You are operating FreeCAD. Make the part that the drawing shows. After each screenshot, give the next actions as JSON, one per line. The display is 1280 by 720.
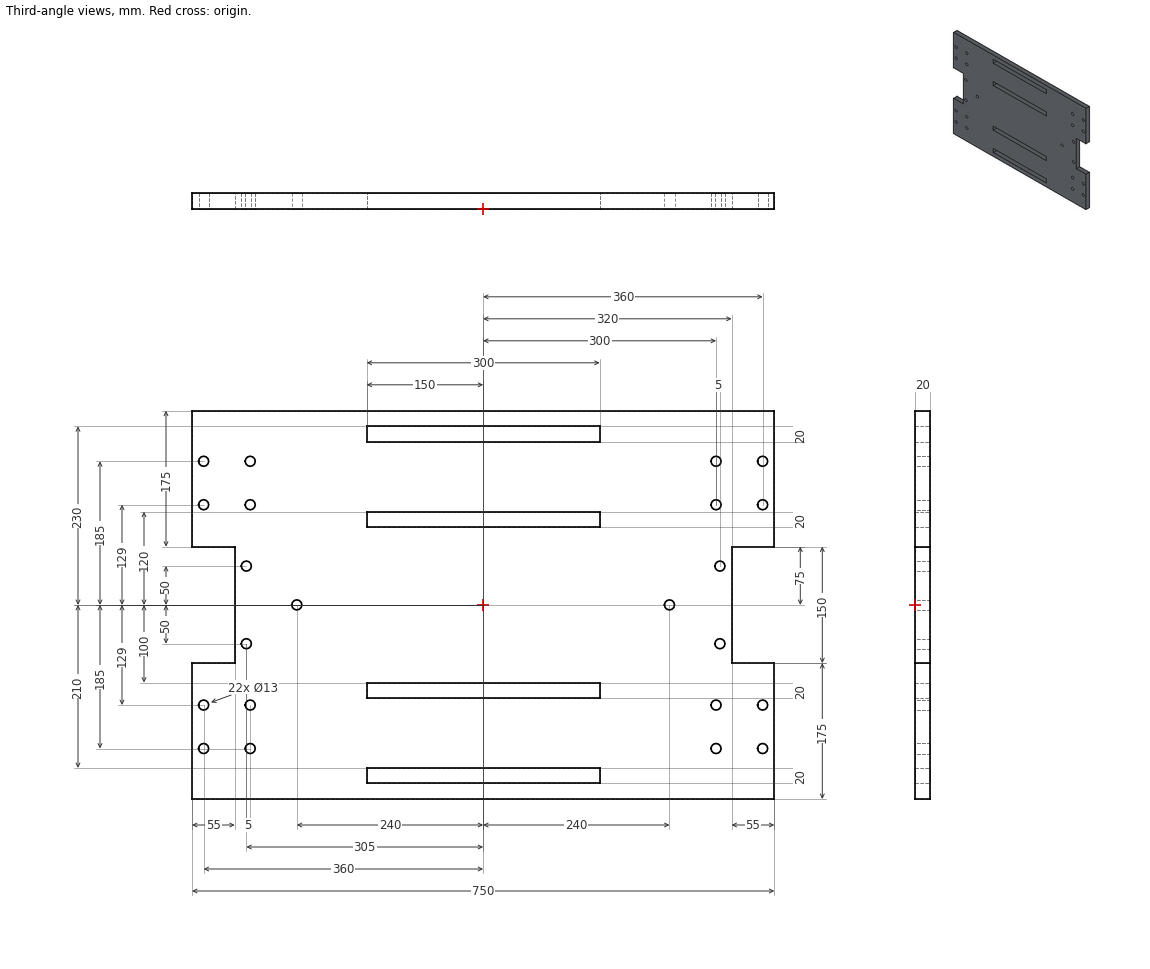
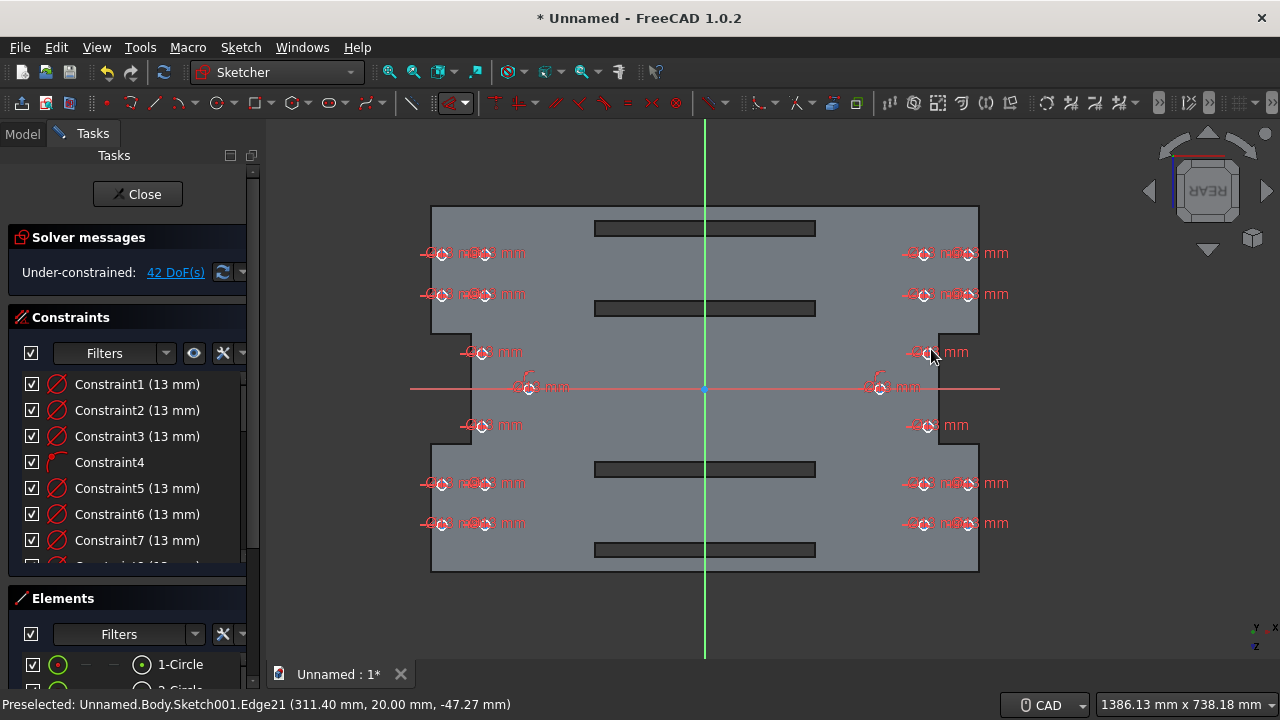
{"action": "left_click", "coordinate": [442, 296]}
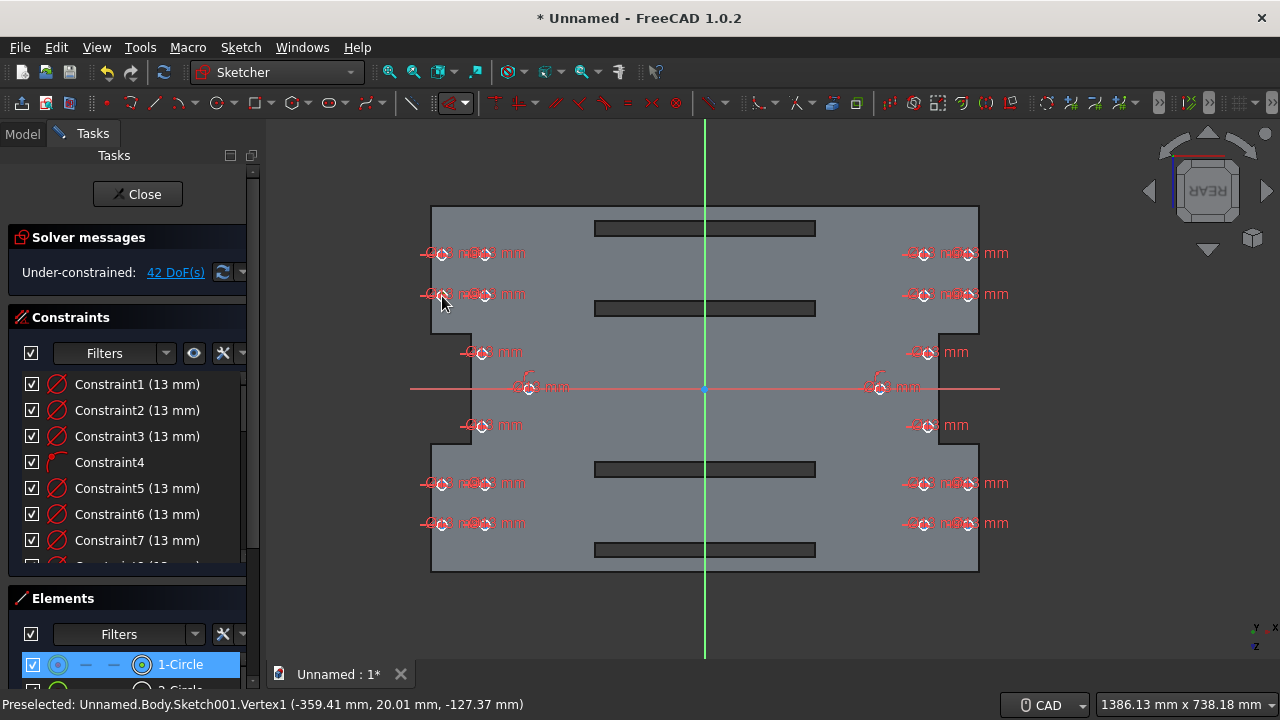
{"action": "left_click", "coordinate": [485, 296]}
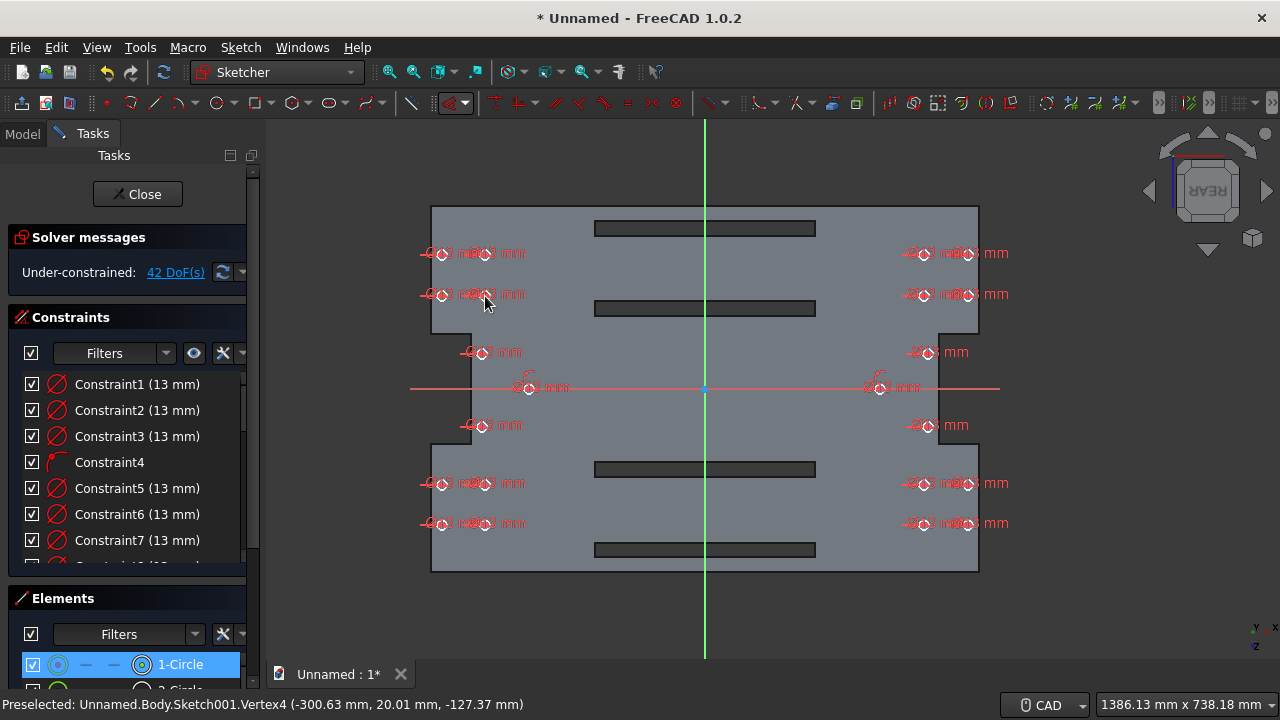
{"action": "left_click", "coordinate": [538, 104]}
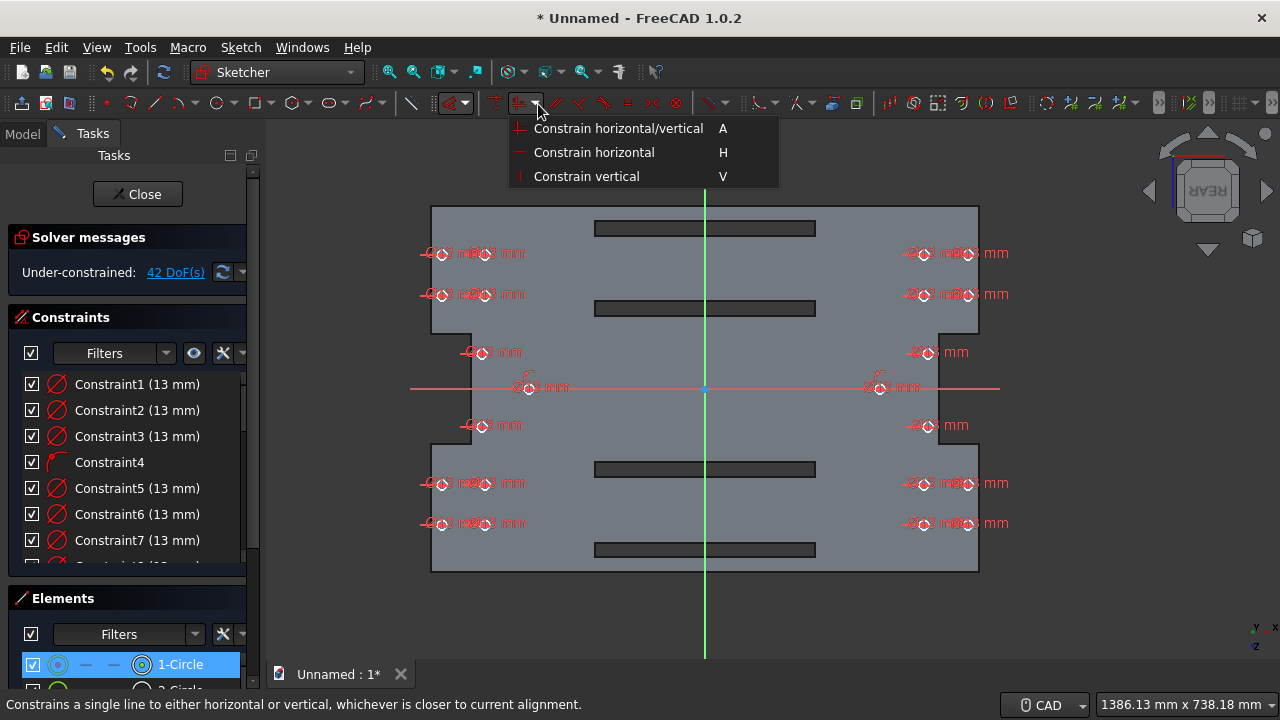
{"action": "left_click", "coordinate": [644, 152]}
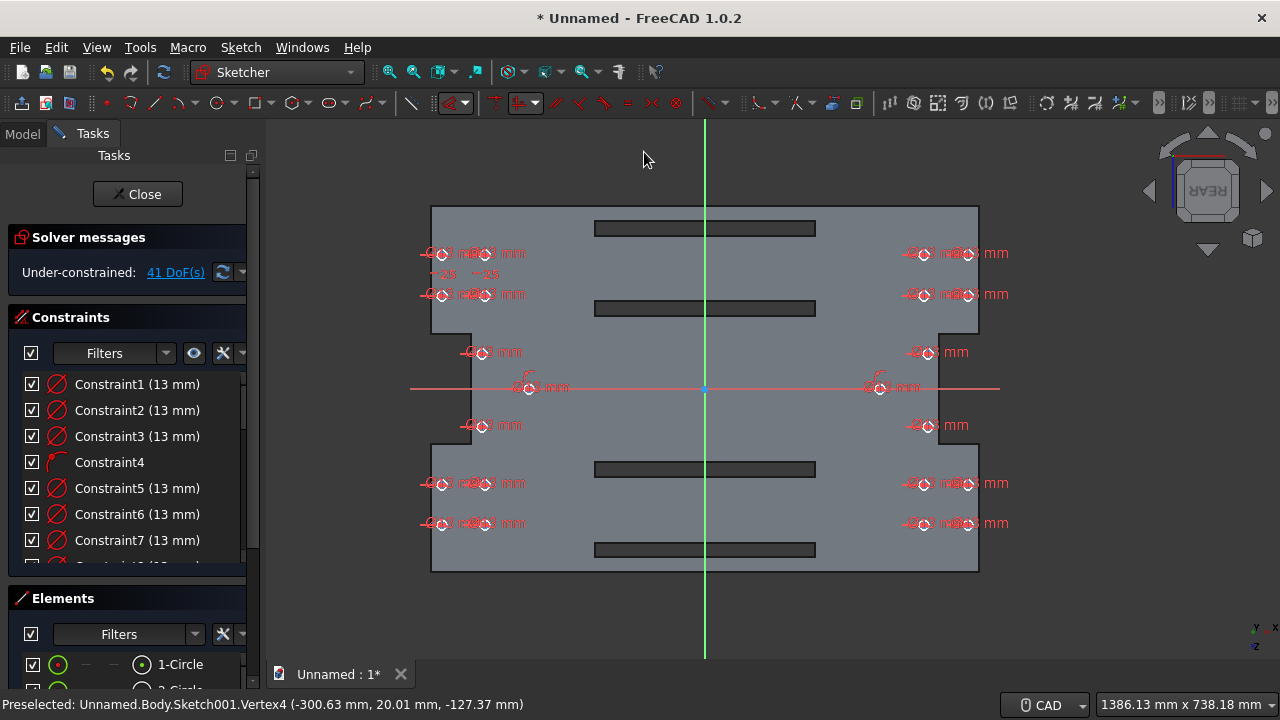
{"action": "left_click", "coordinate": [485, 296]}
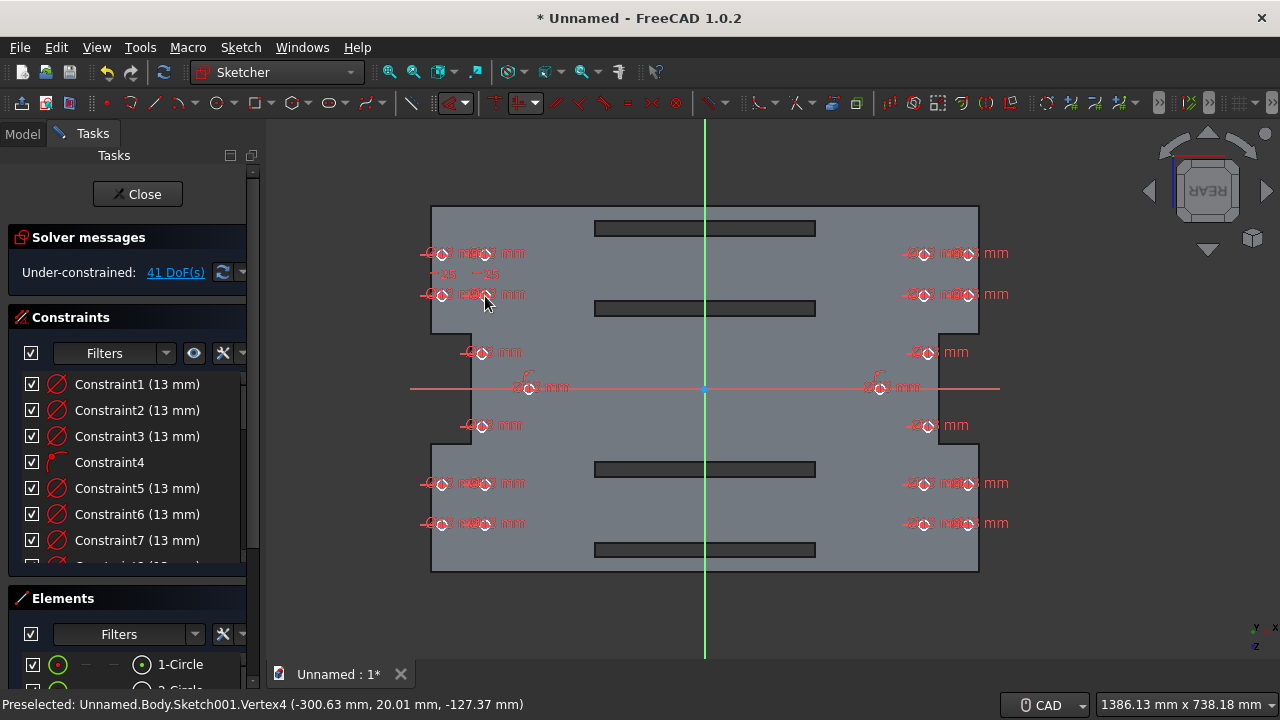
{"action": "left_click", "coordinate": [485, 255]}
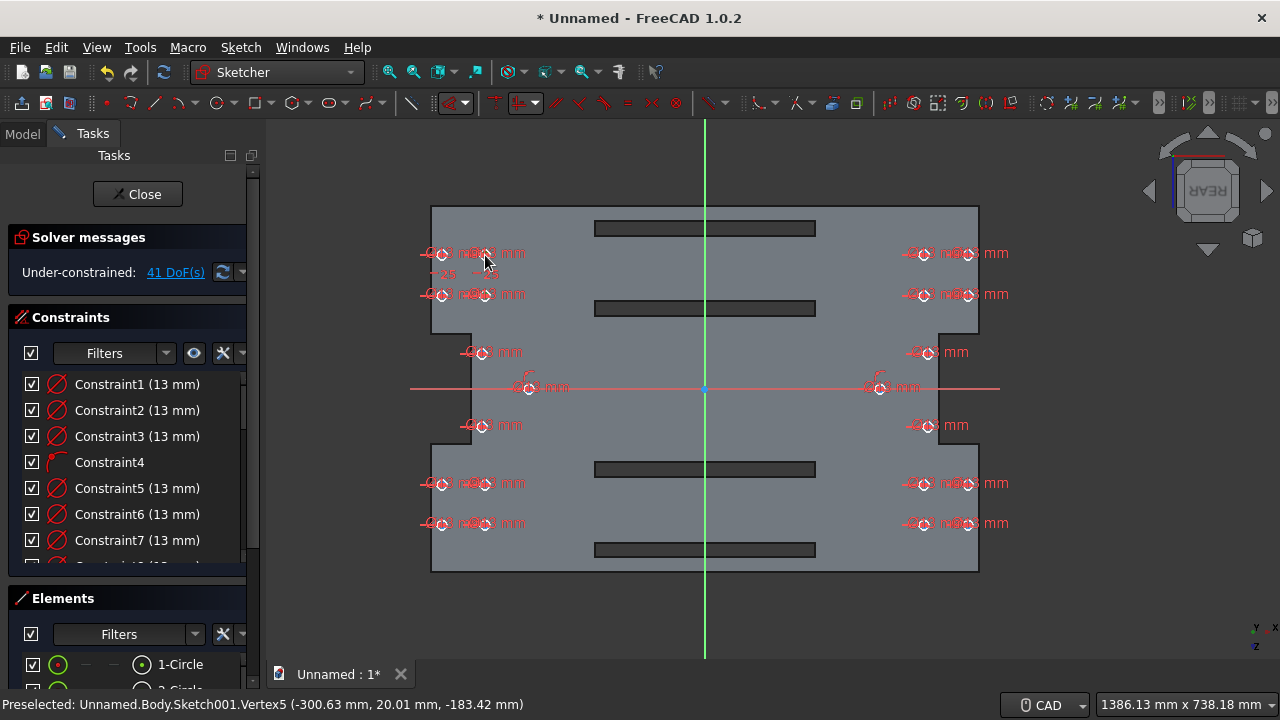
{"action": "key", "text": "v"}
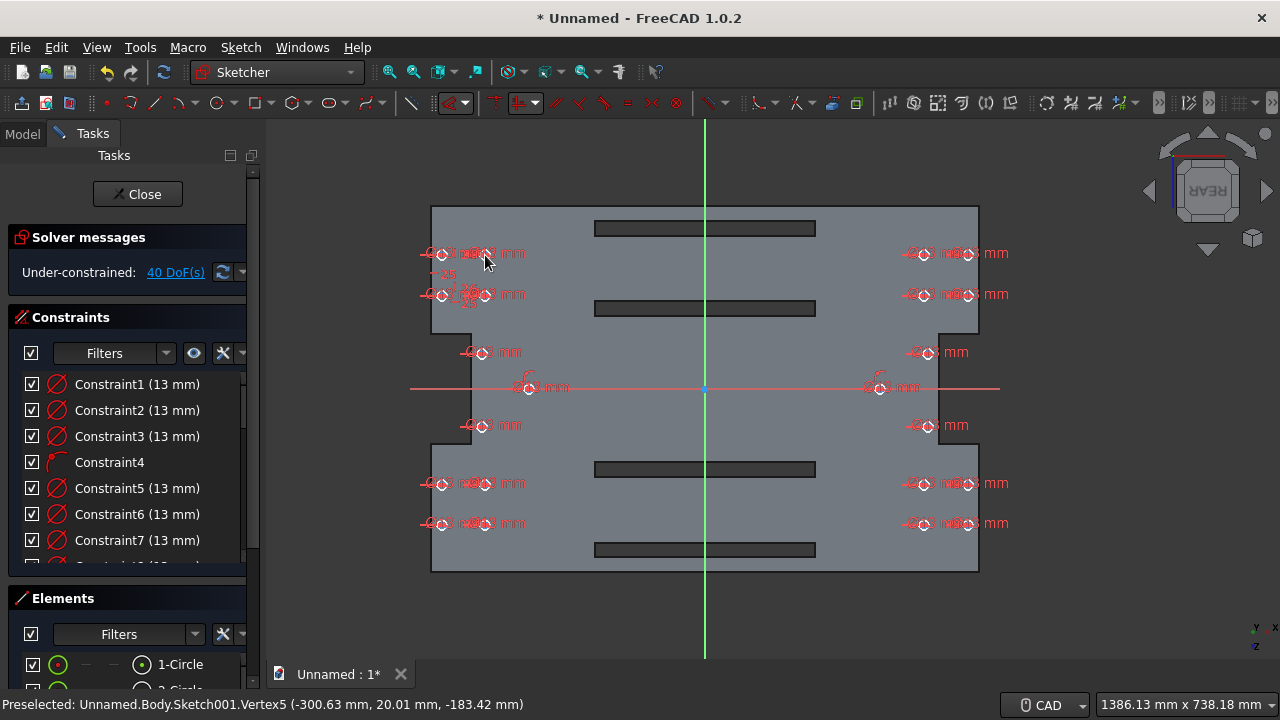
{"action": "left_click", "coordinate": [442, 296]}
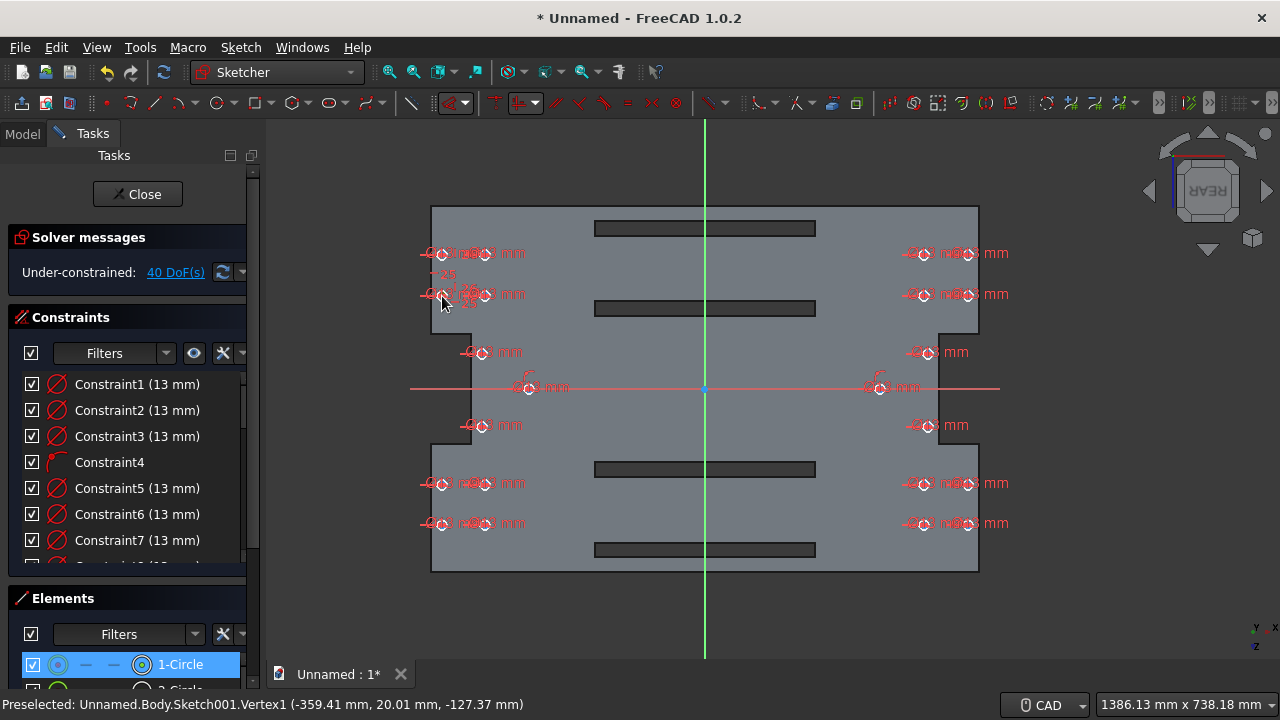
{"action": "left_click", "coordinate": [442, 255]}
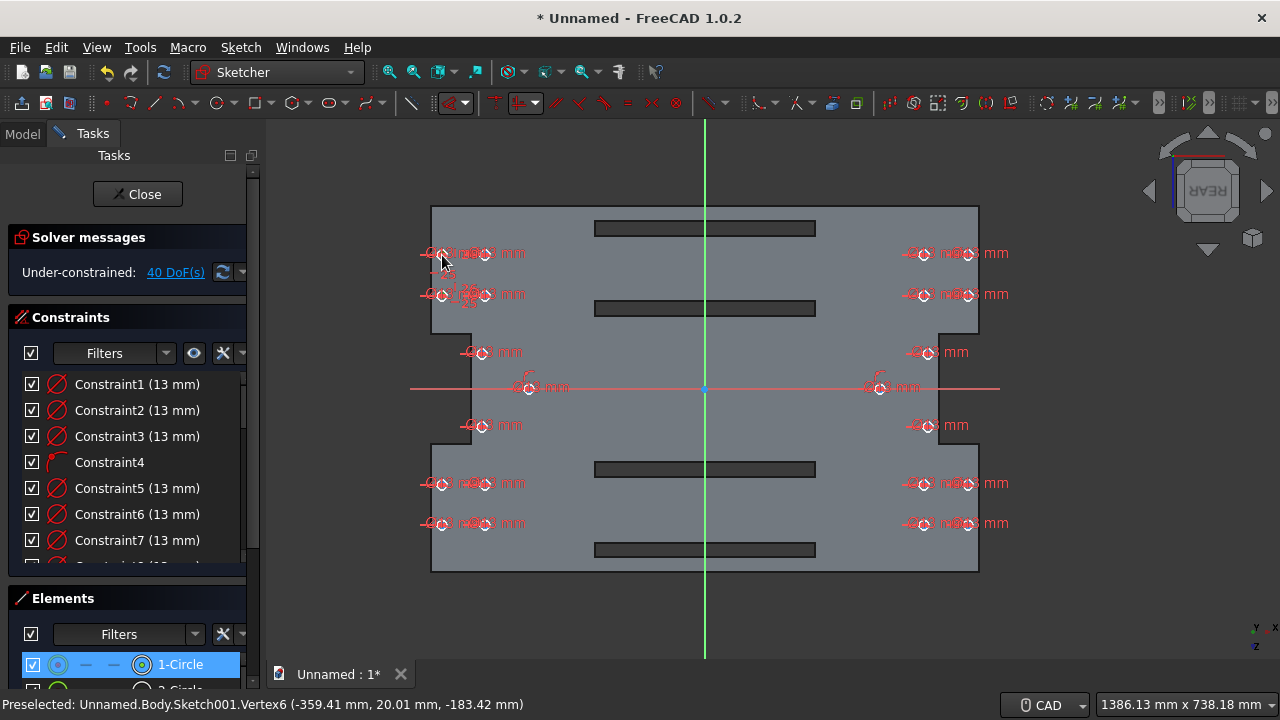
{"action": "key", "text": "v"}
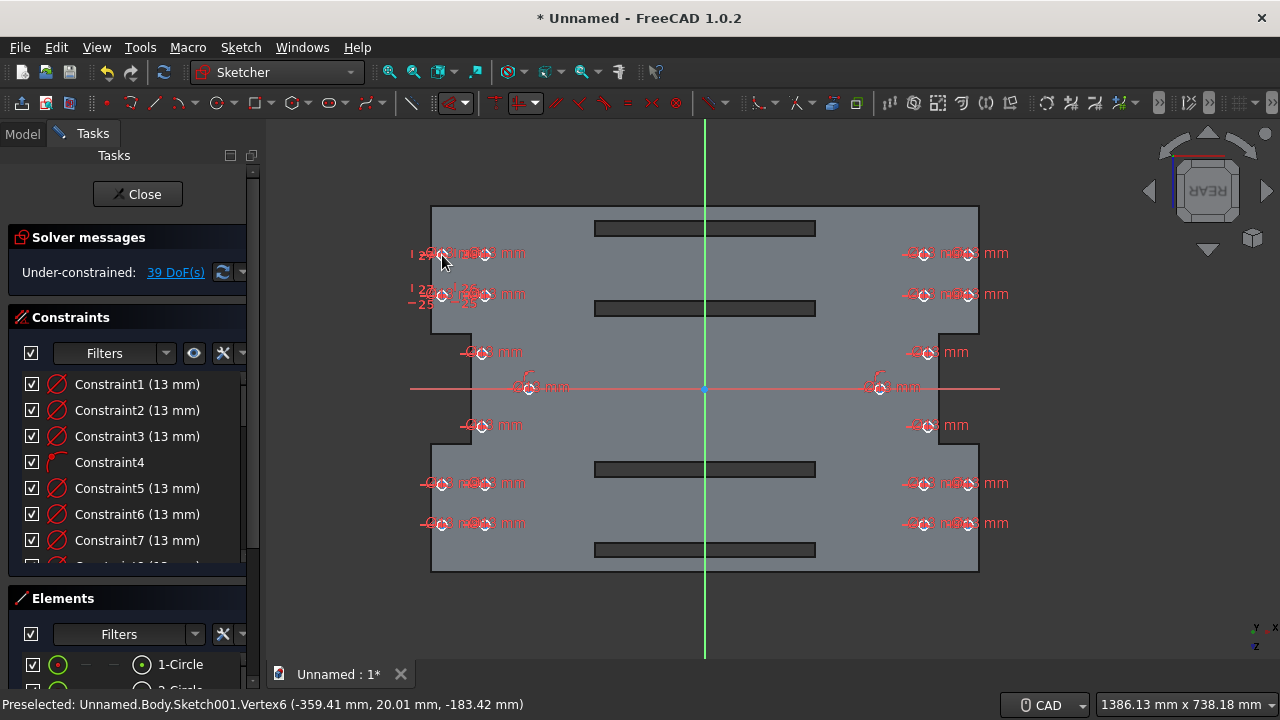
{"action": "left_click", "coordinate": [485, 255]}